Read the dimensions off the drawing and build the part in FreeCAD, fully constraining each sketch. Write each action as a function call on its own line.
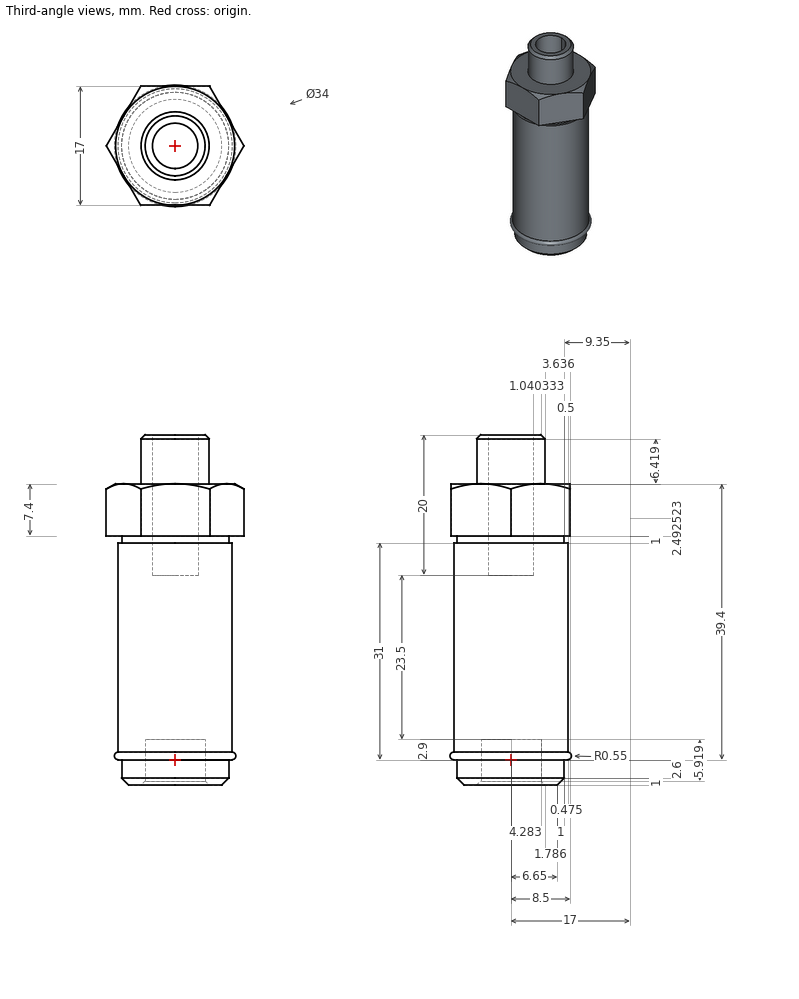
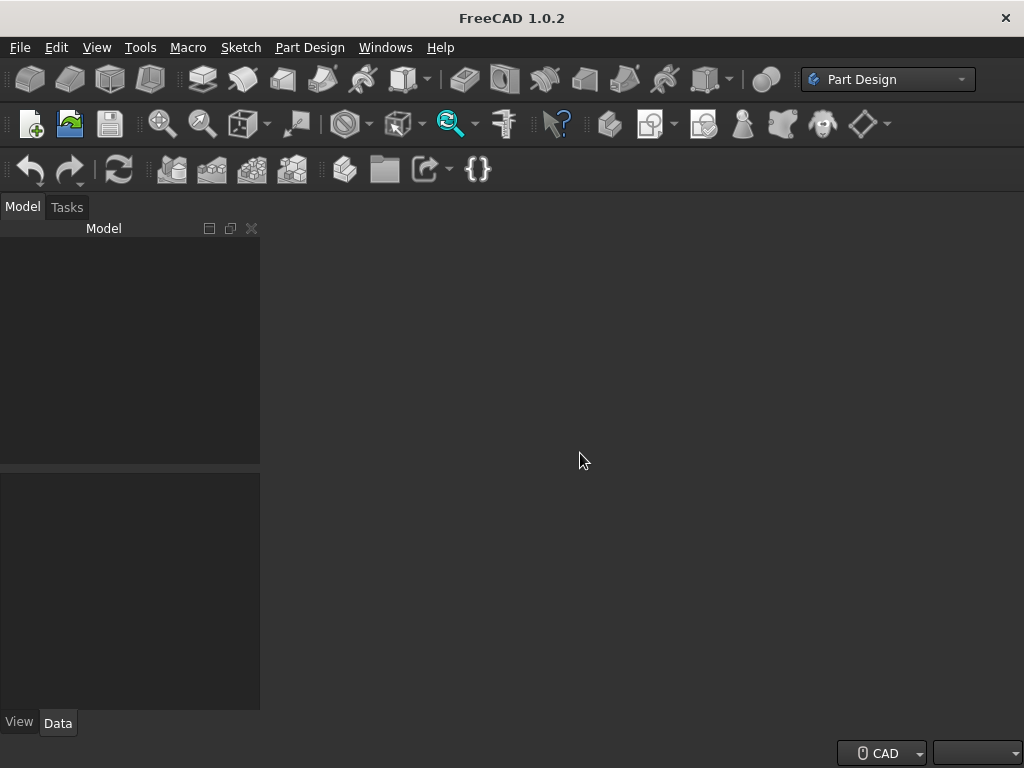
key(ctrl+n)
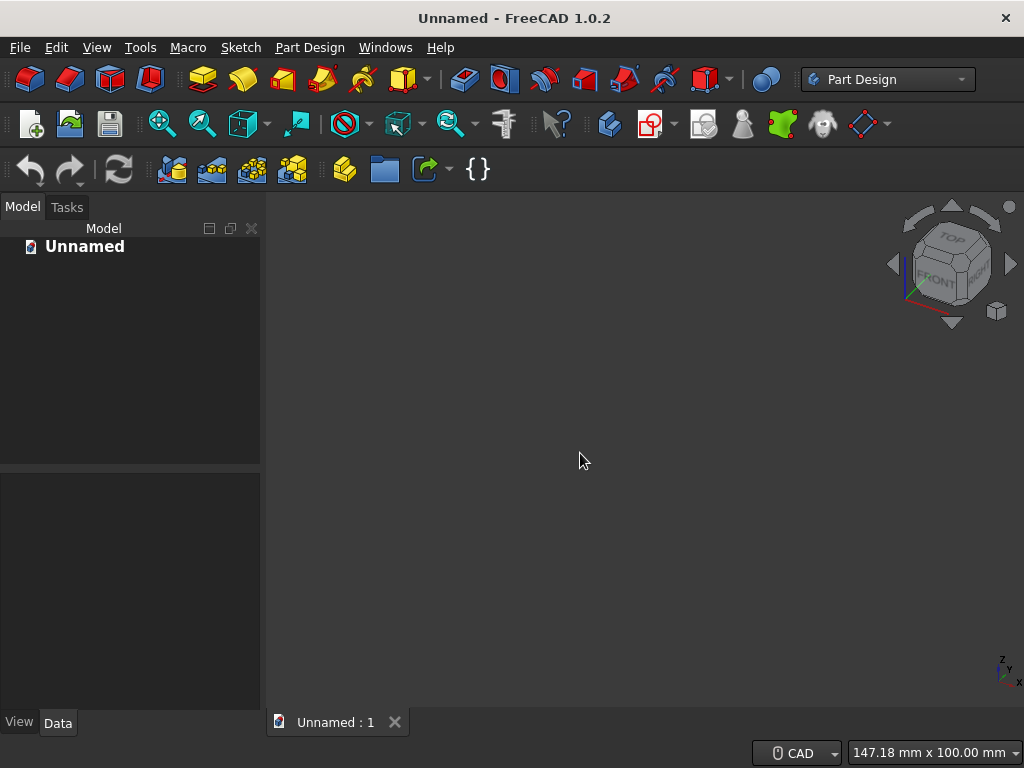
click(650, 124)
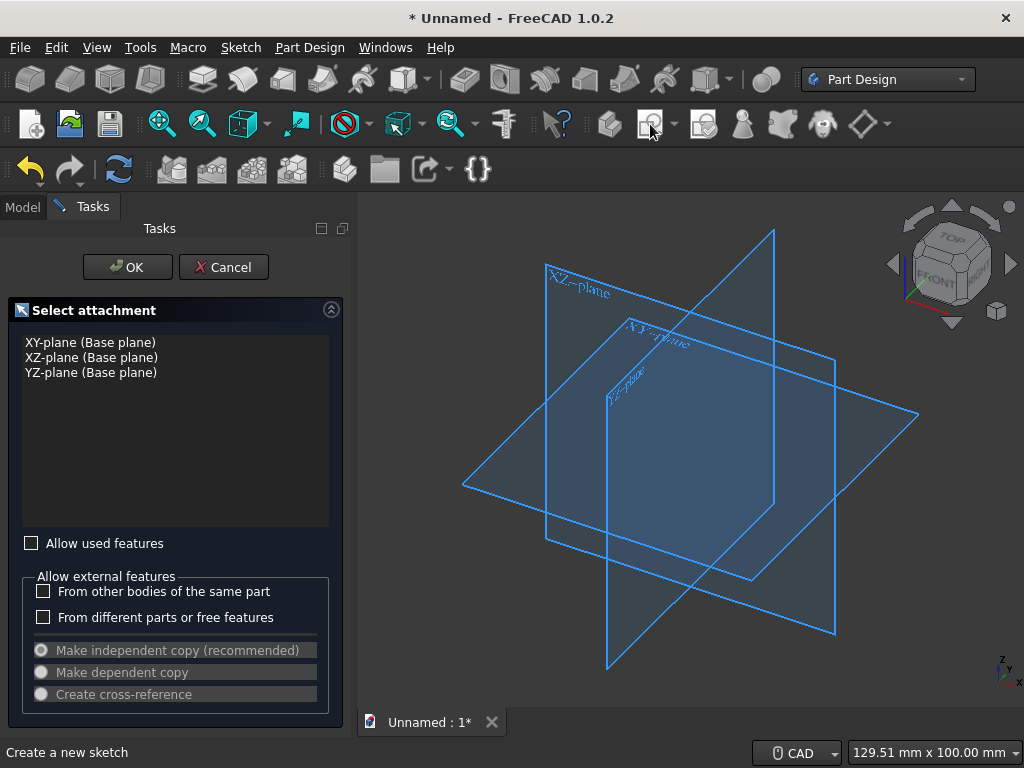
click(82, 372)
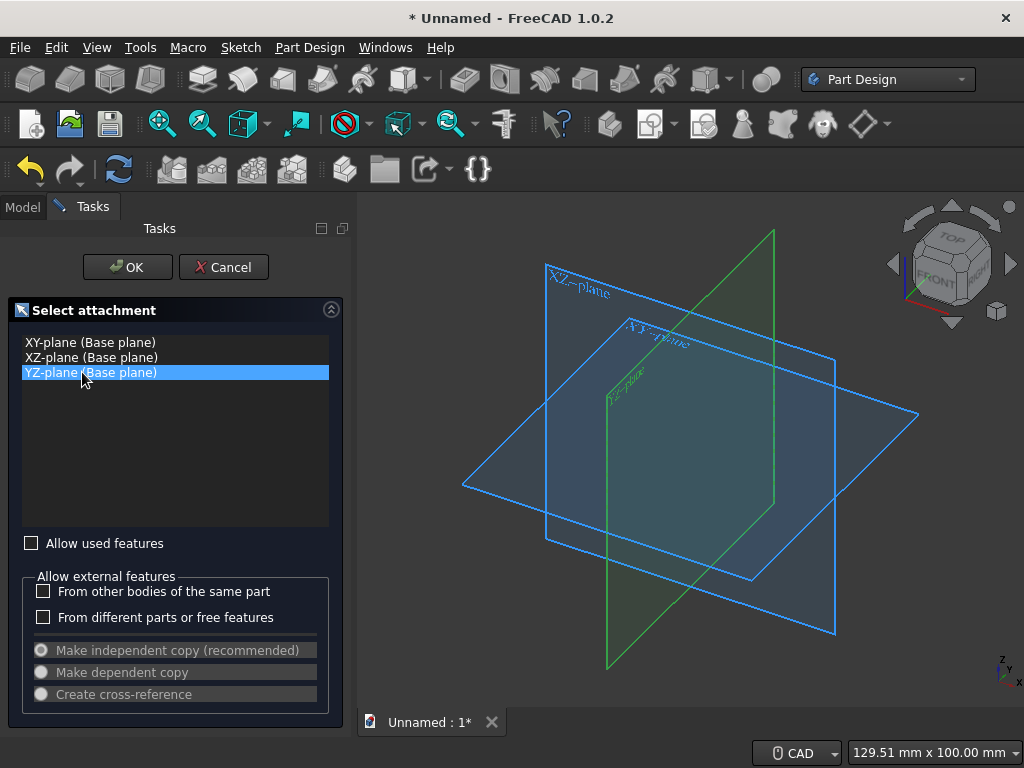
click(128, 267)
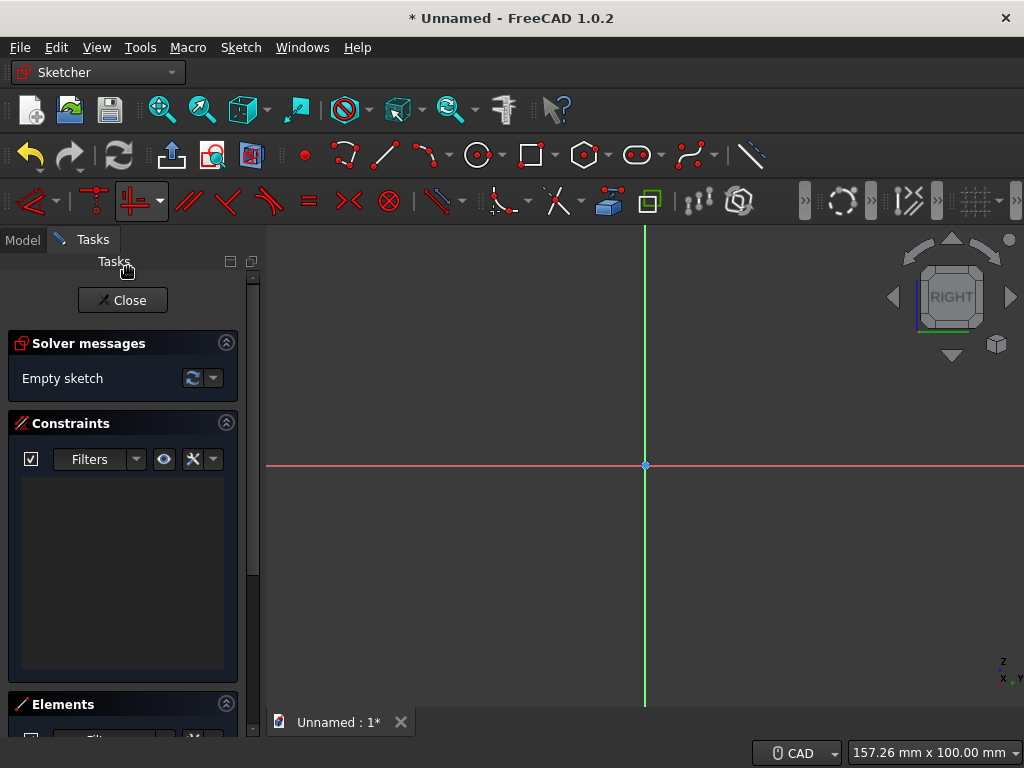
scroll(294, 679, down, 1)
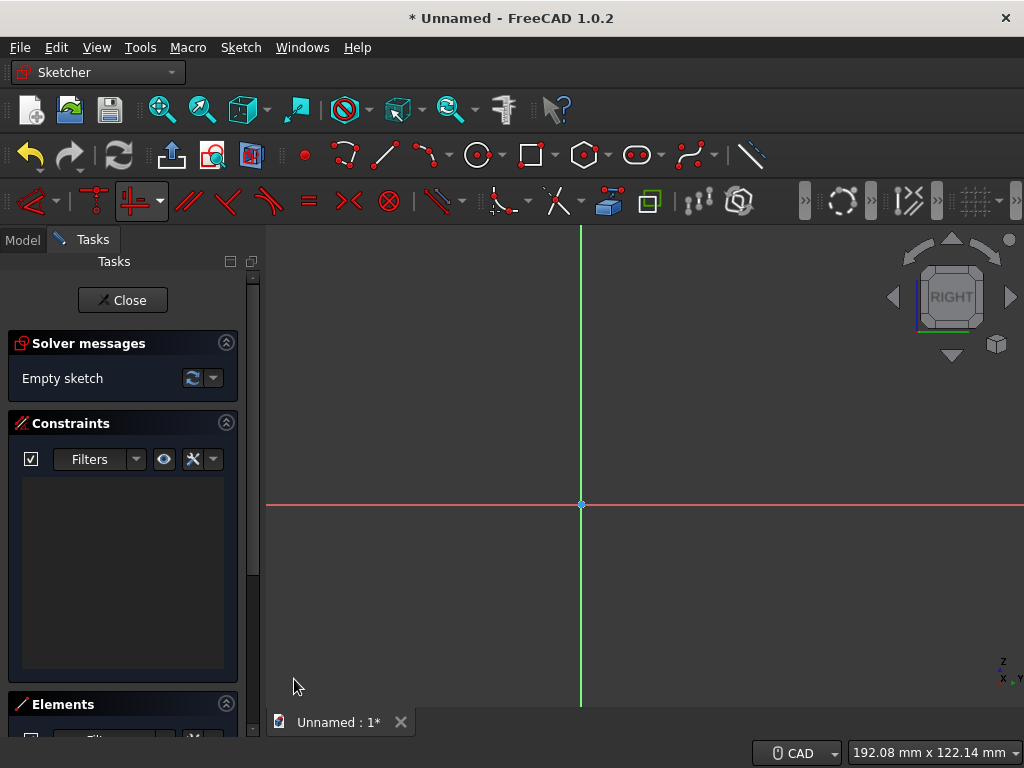
scroll(693, 327, up, 2)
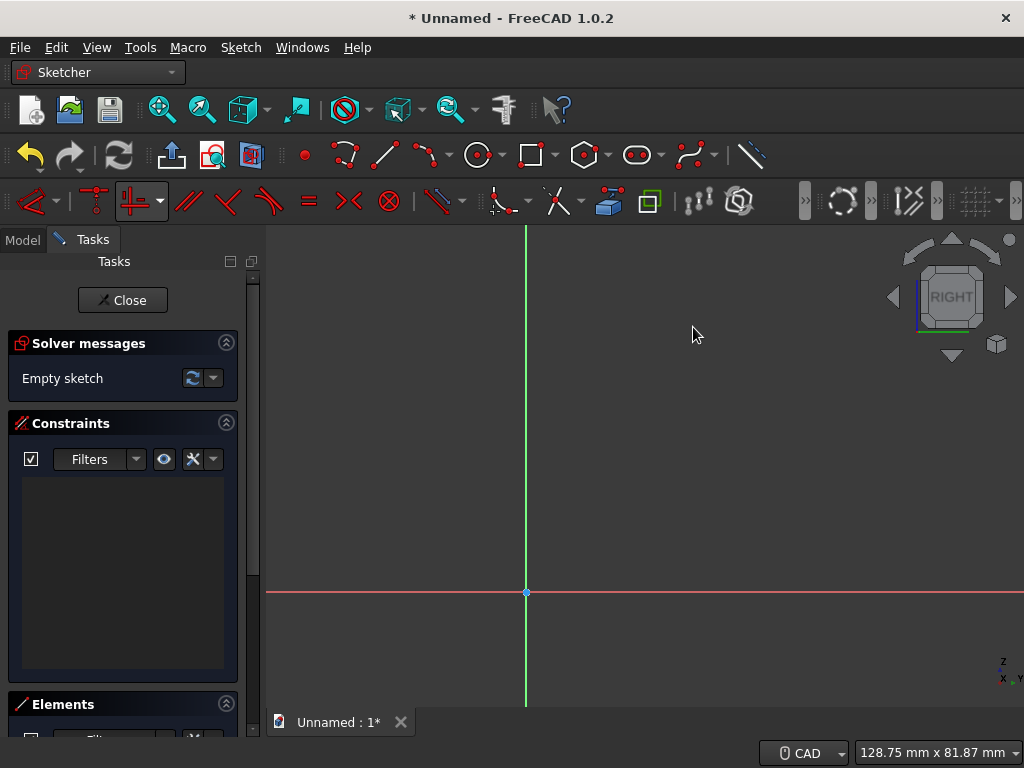
key(g)
key(m)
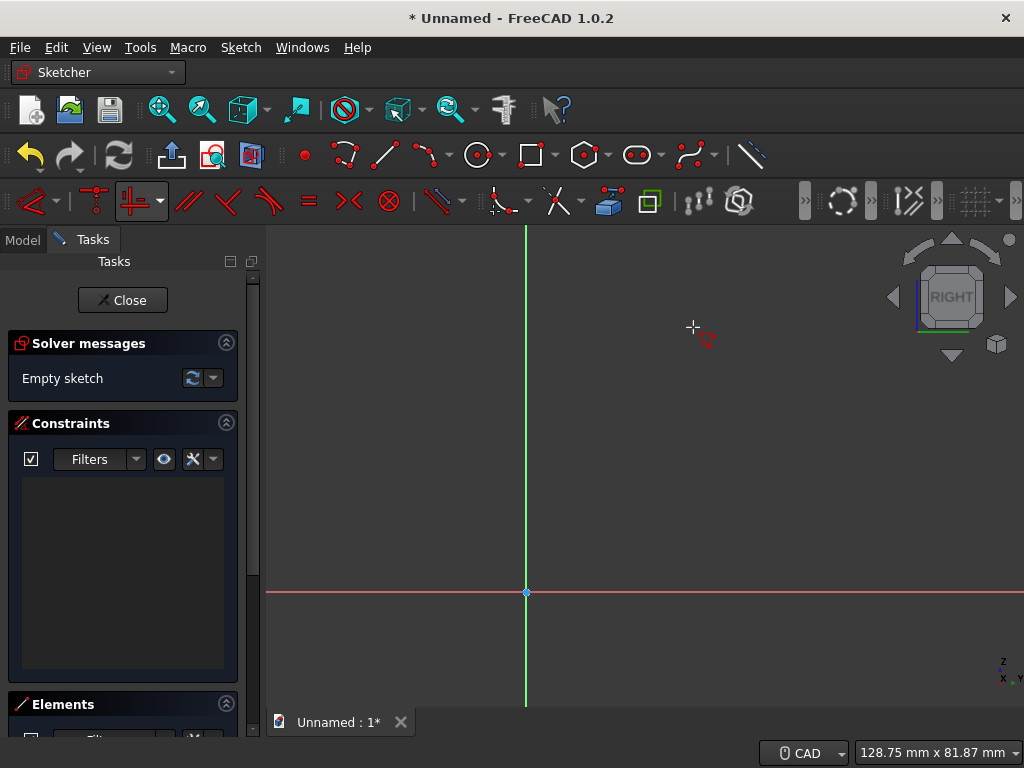
scroll(574, 586, up, 5)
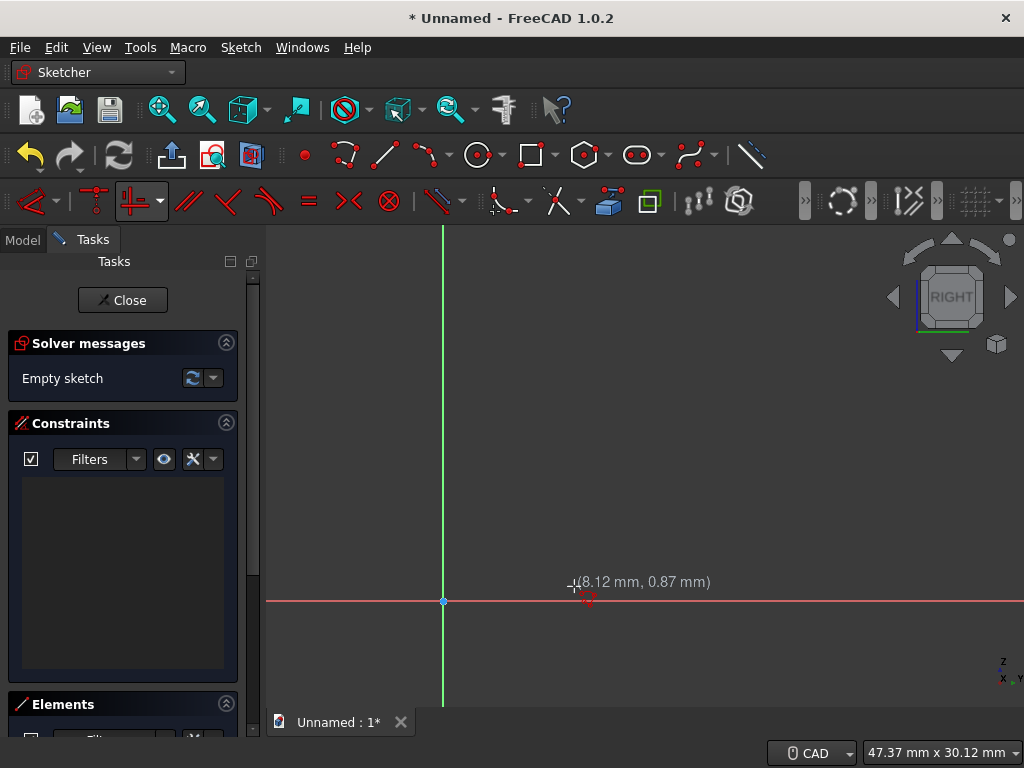
click(574, 584)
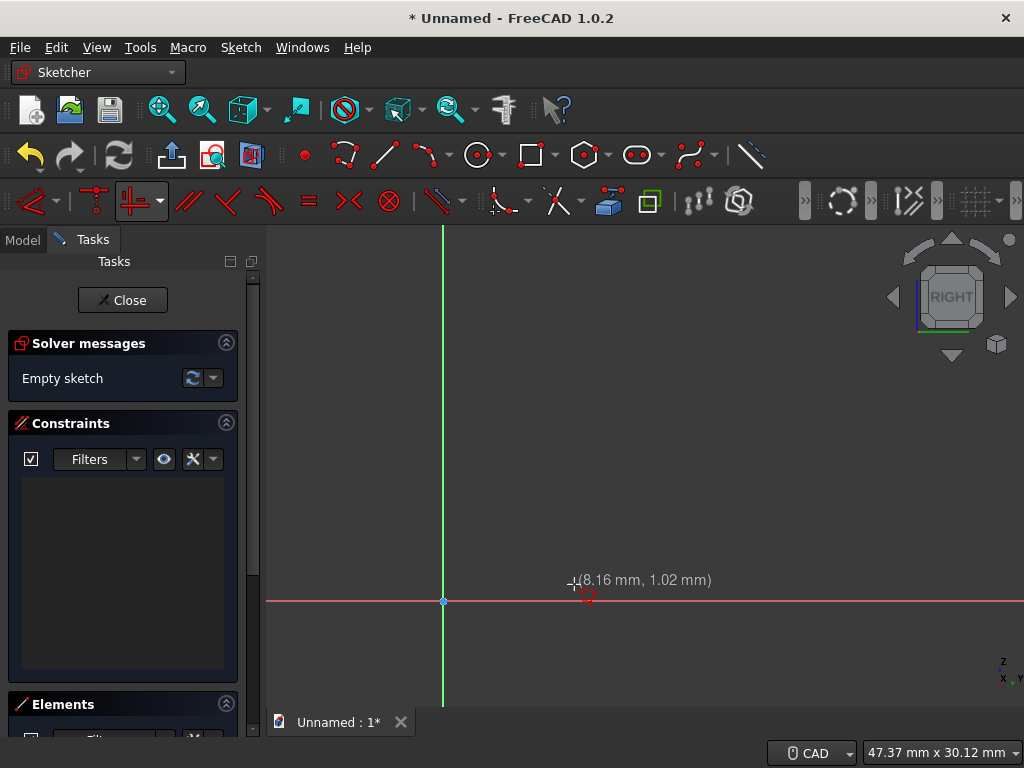
scroll(575, 587, down, 5)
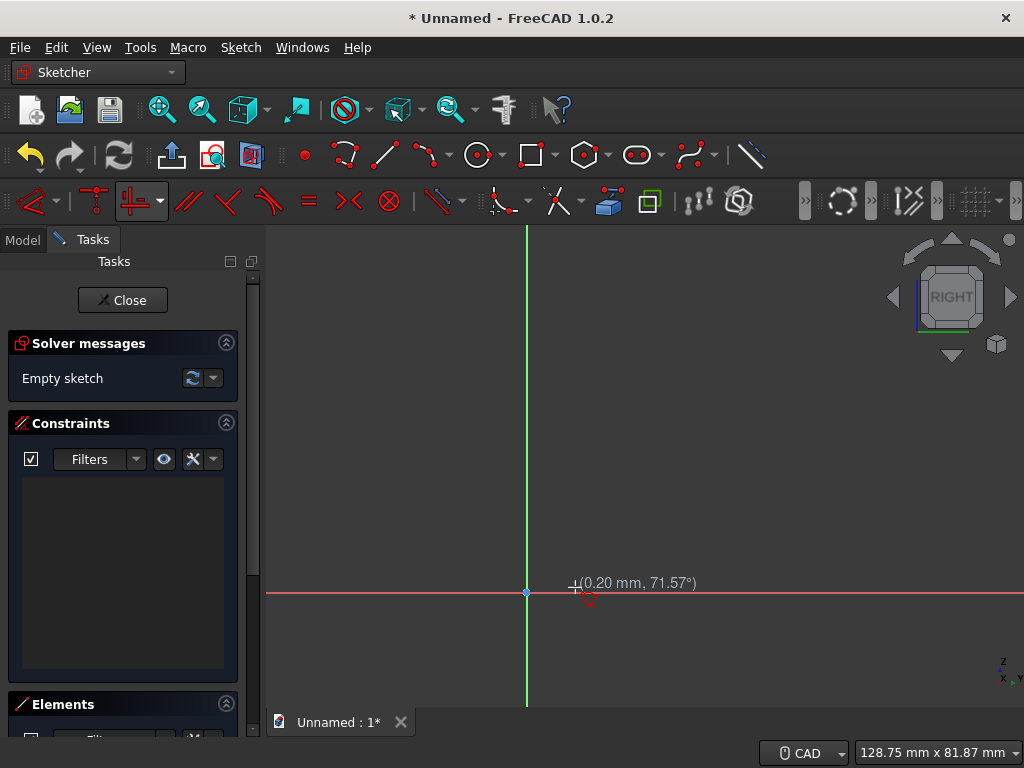
click(575, 410)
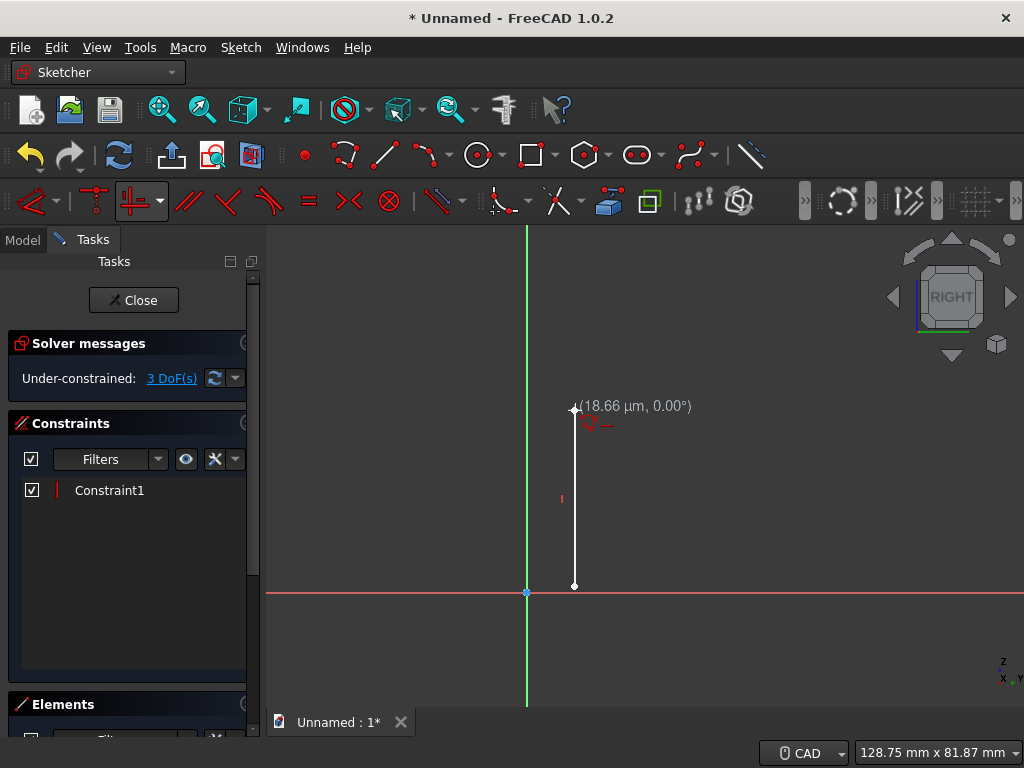
scroll(572, 410, up, 9)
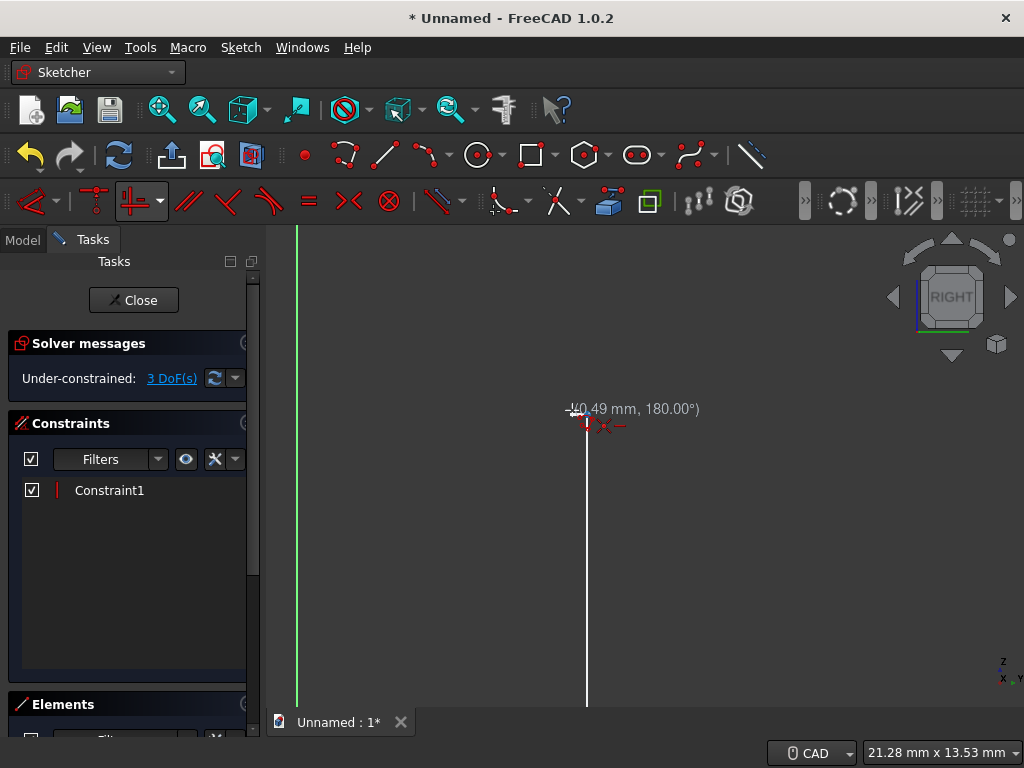
click(569, 408)
click(569, 374)